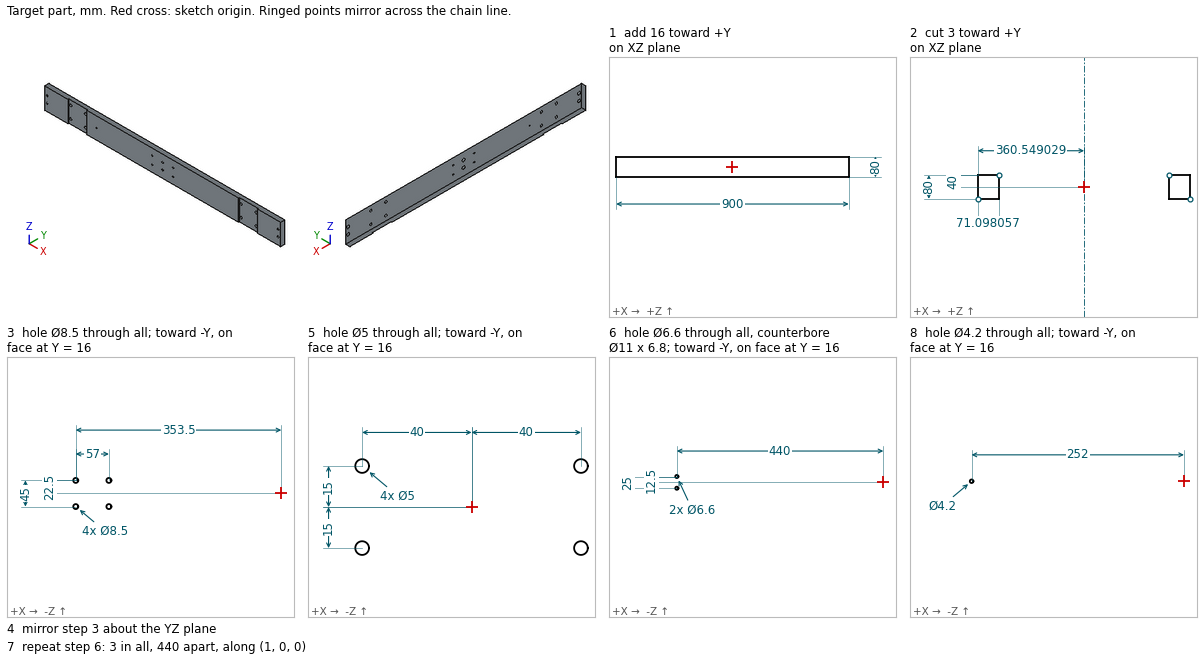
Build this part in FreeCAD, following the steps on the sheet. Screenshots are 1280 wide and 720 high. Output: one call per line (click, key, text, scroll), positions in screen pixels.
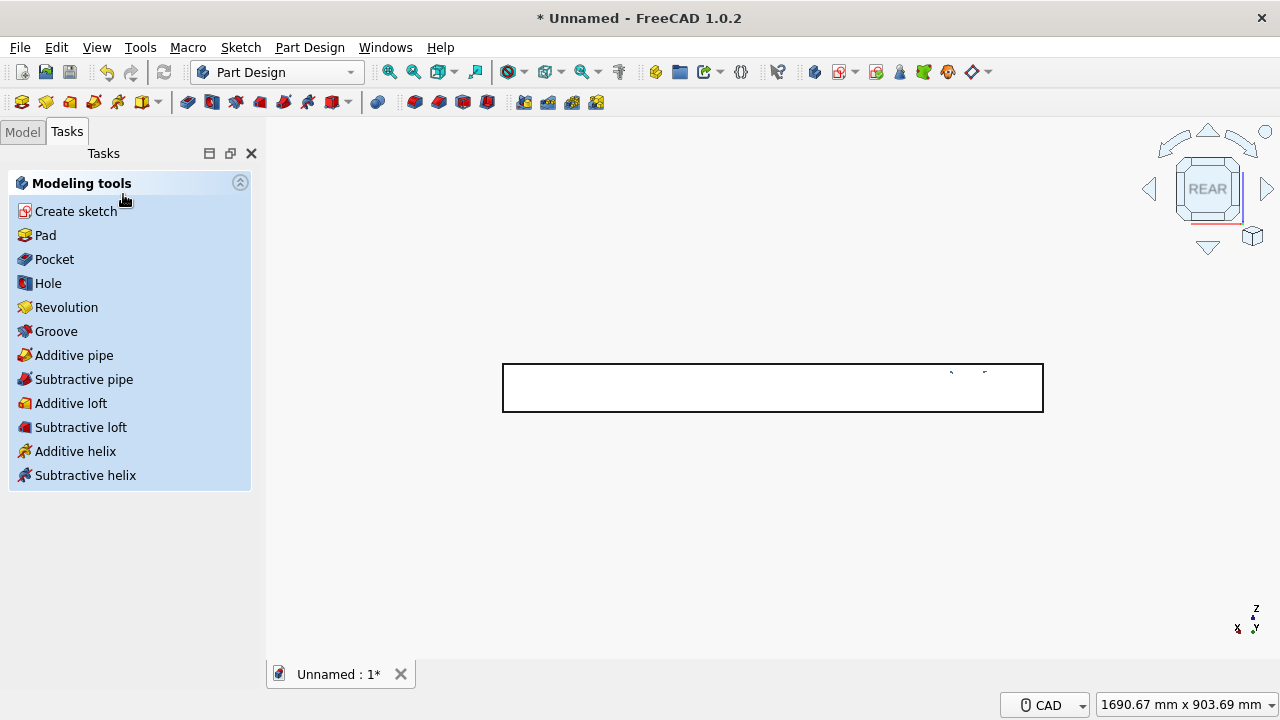
click(212, 102)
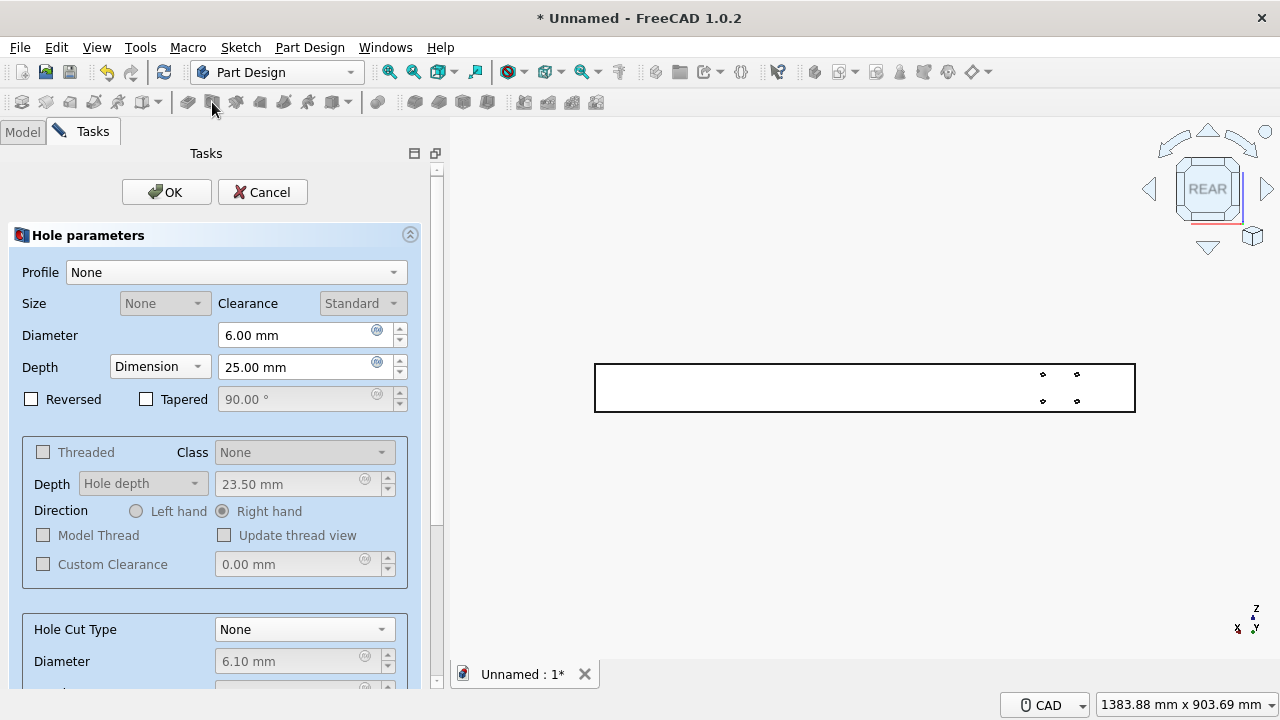
triple_click(305, 335)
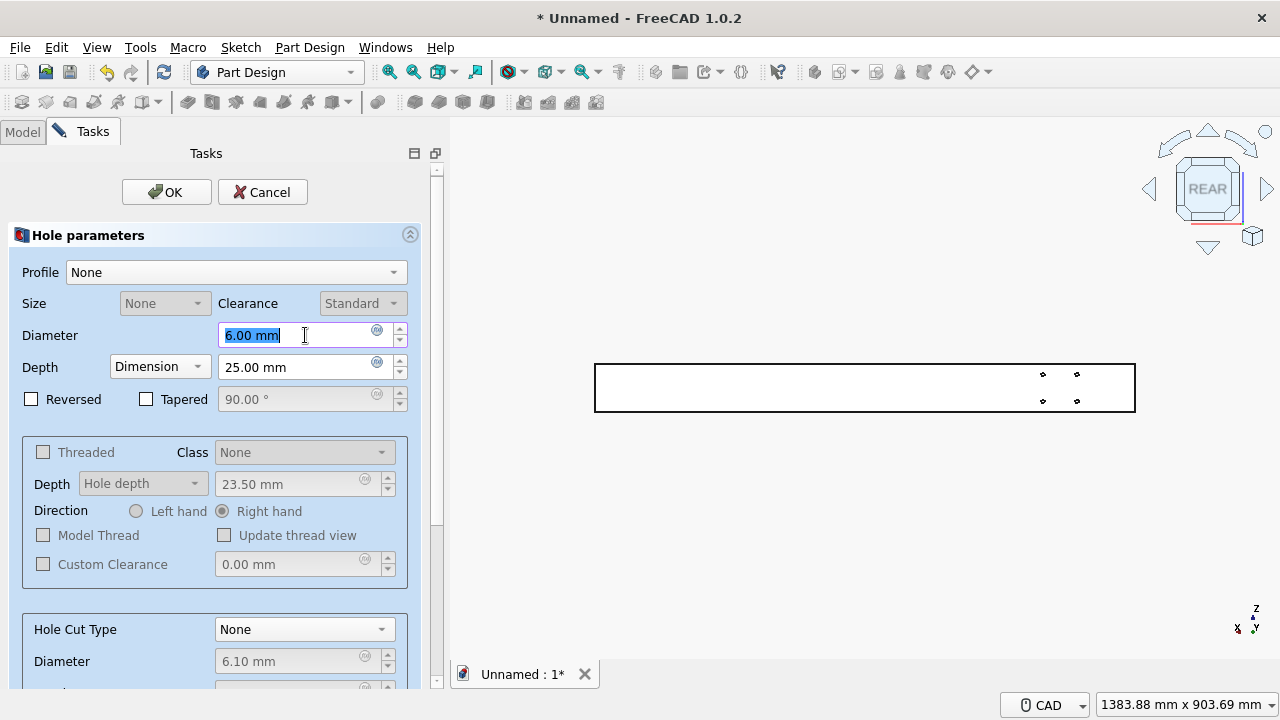
text(8.5)
key(Tab)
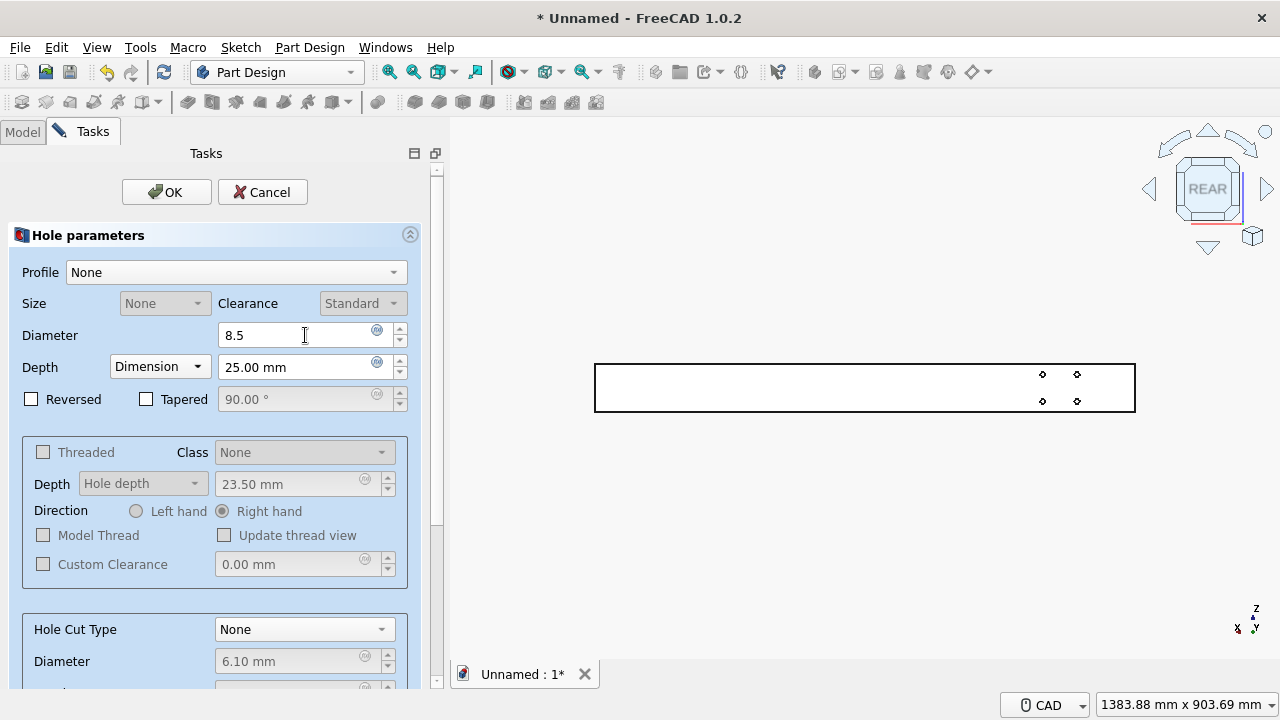
click(161, 366)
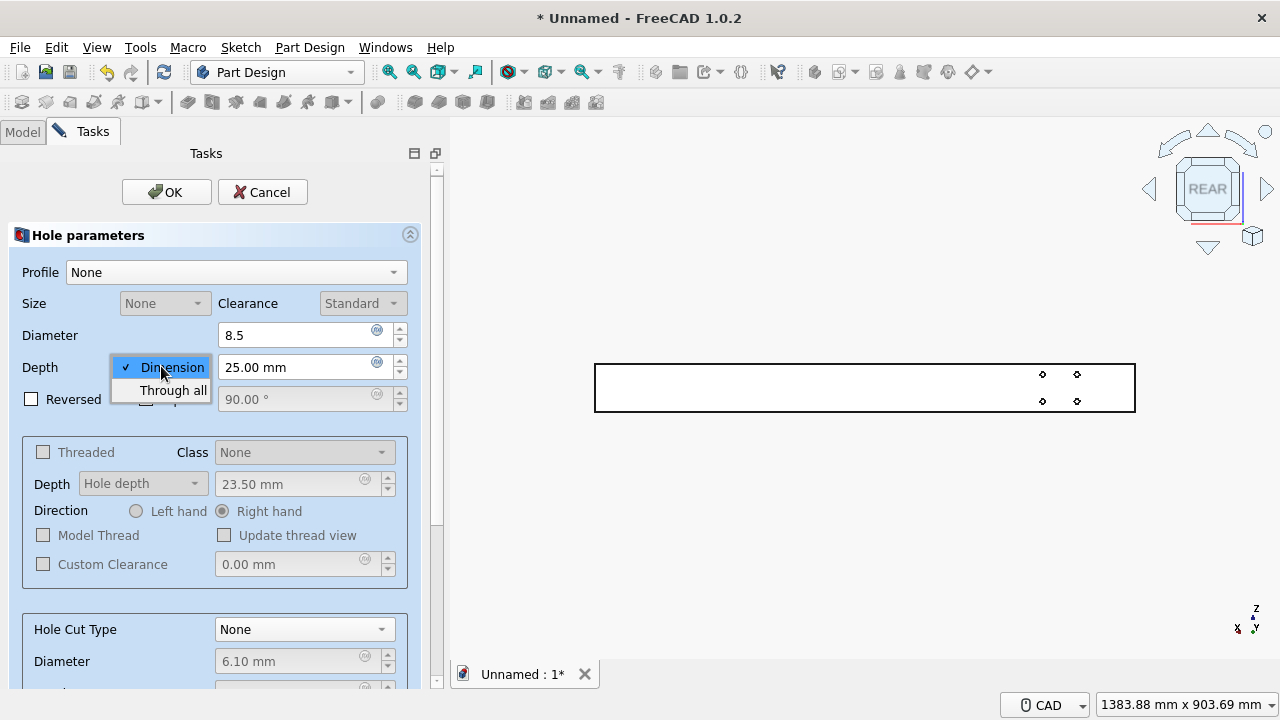
click(160, 390)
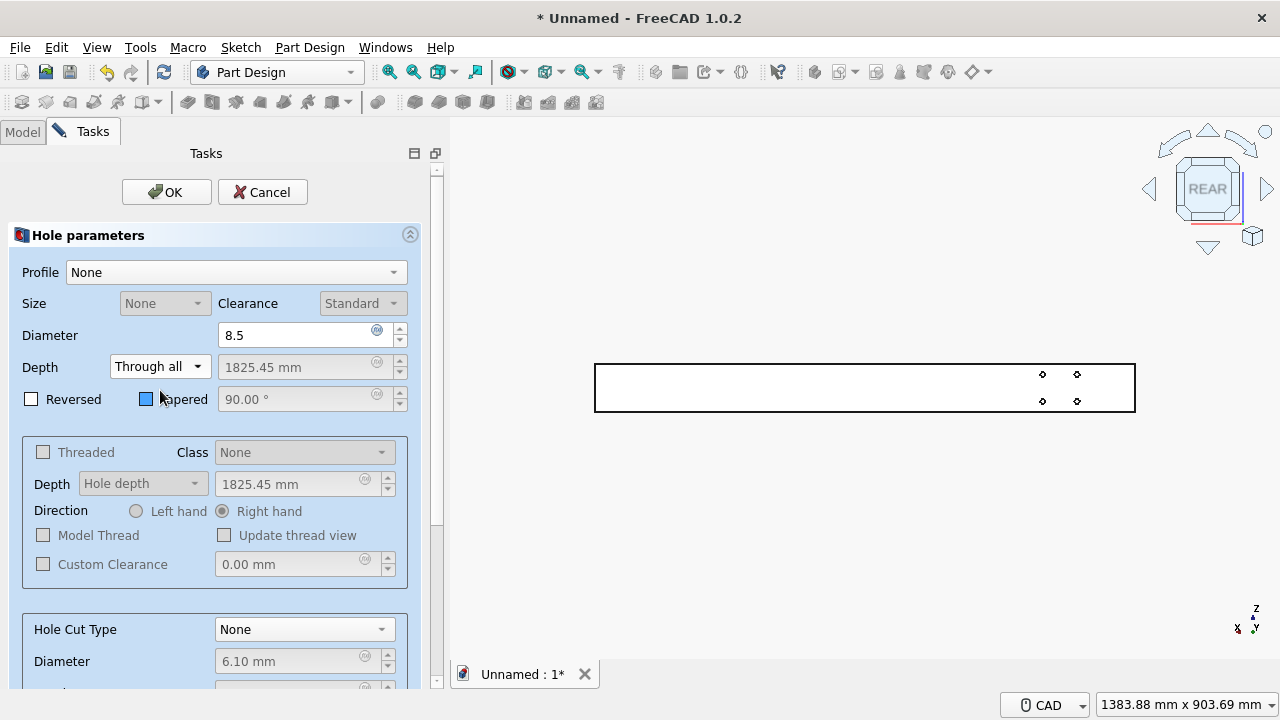
click(167, 192)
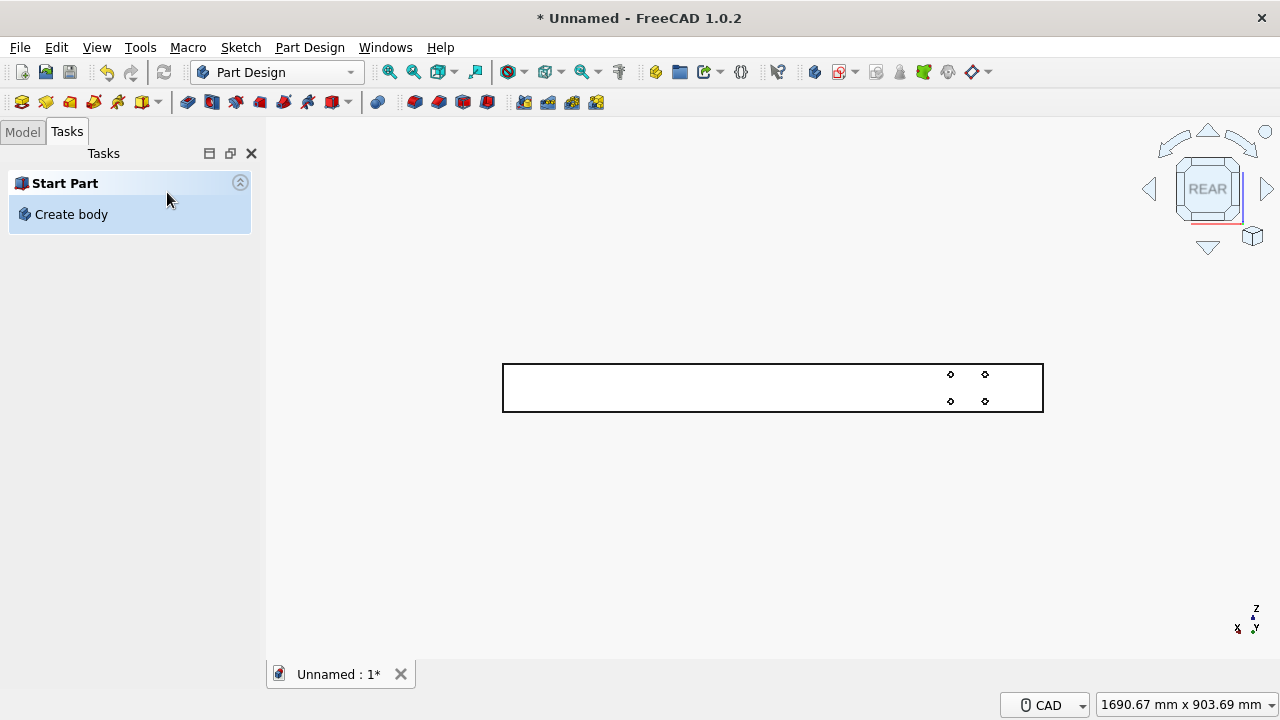
click(23, 131)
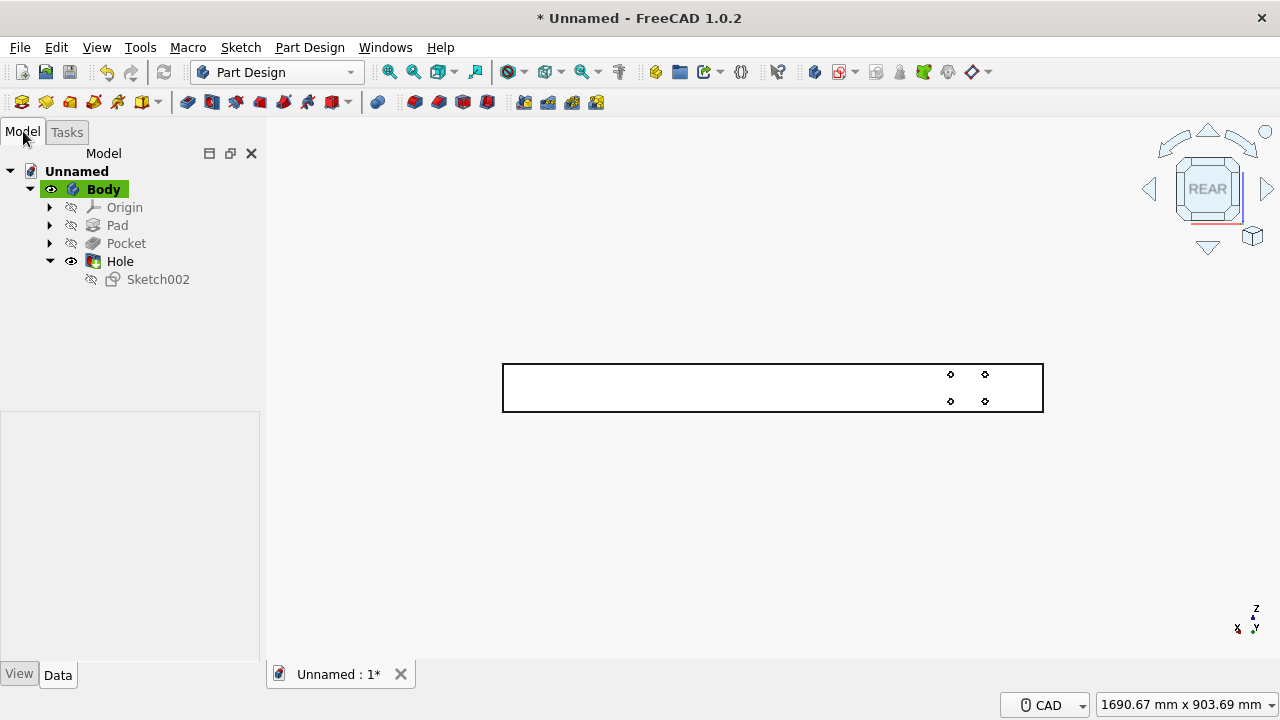
click(116, 261)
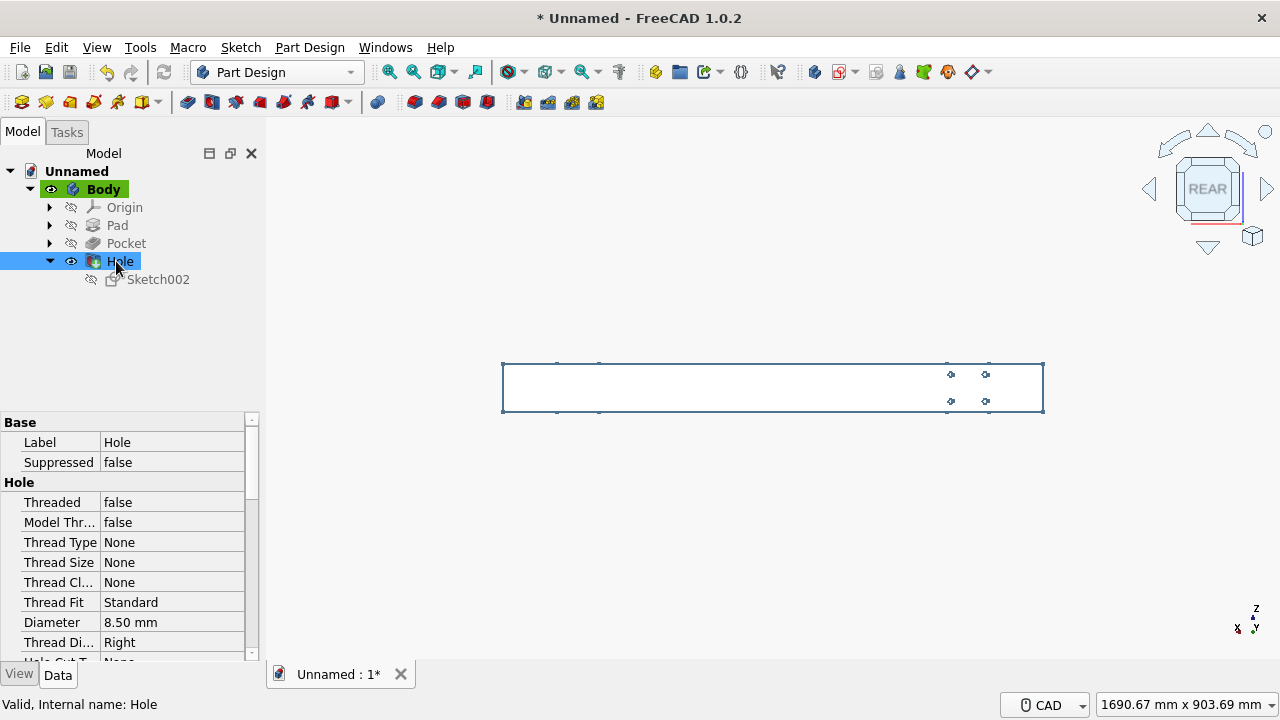
click(524, 102)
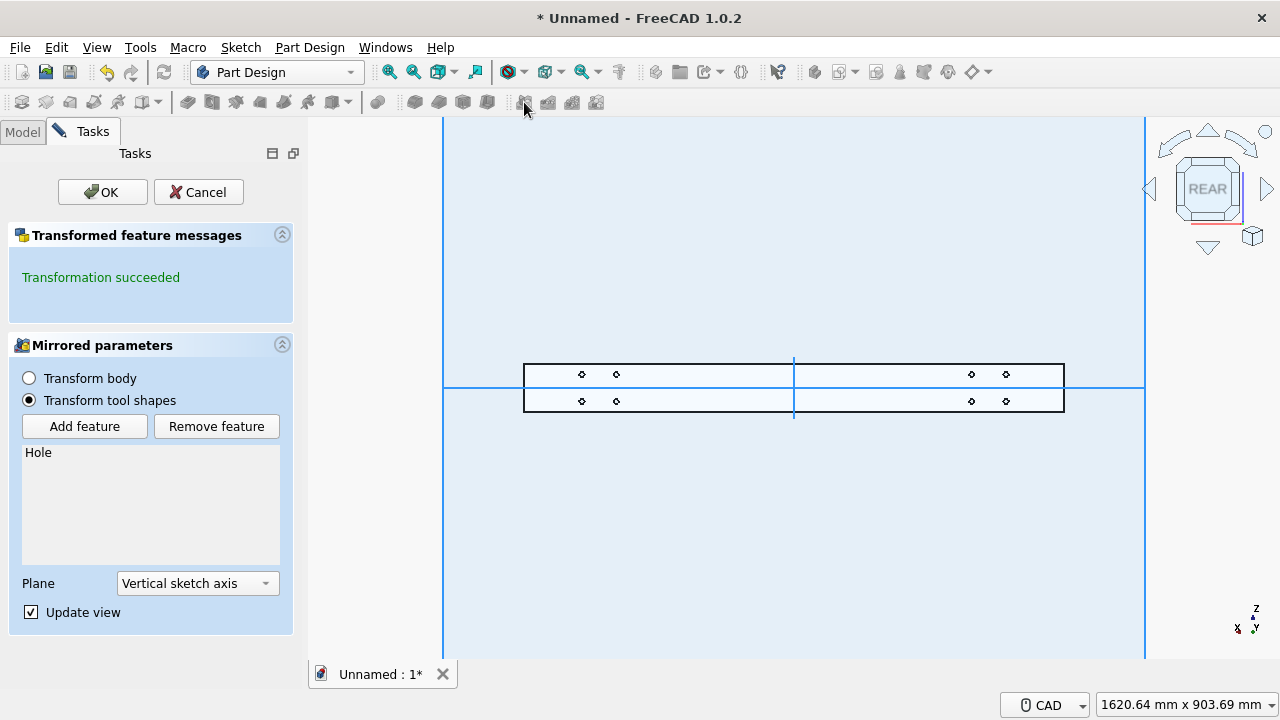
click(198, 584)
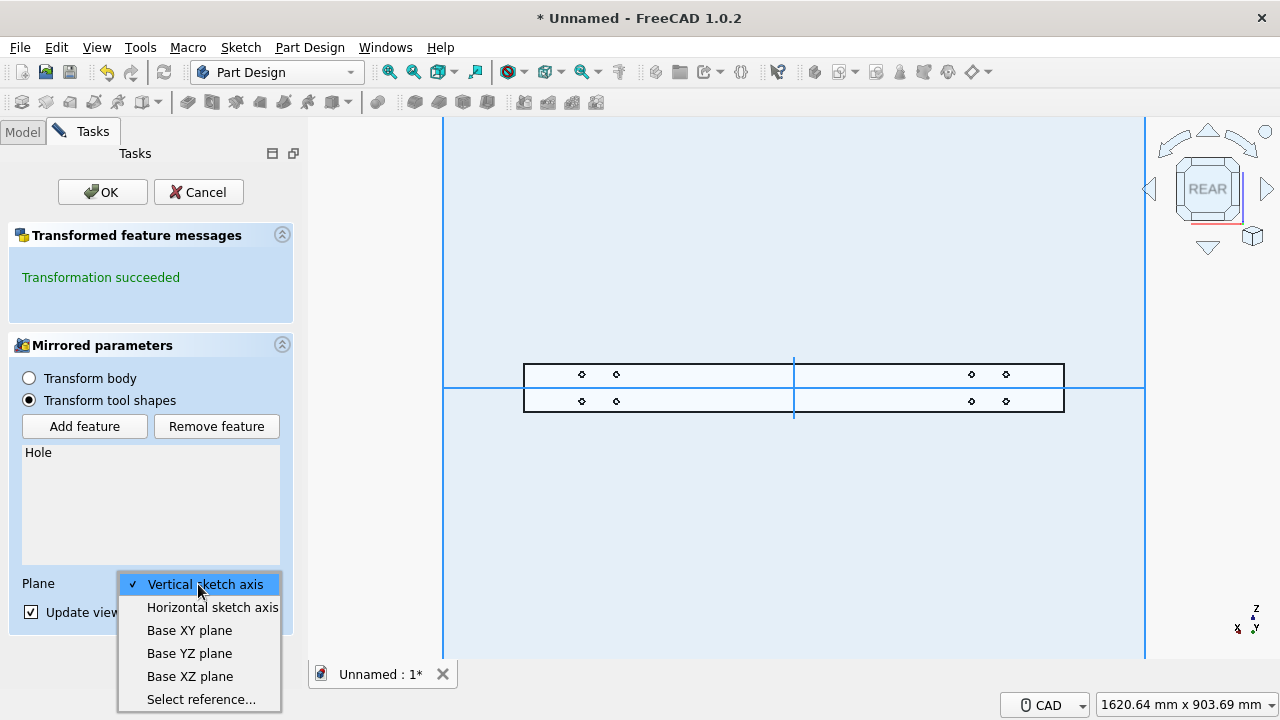
click(198, 654)